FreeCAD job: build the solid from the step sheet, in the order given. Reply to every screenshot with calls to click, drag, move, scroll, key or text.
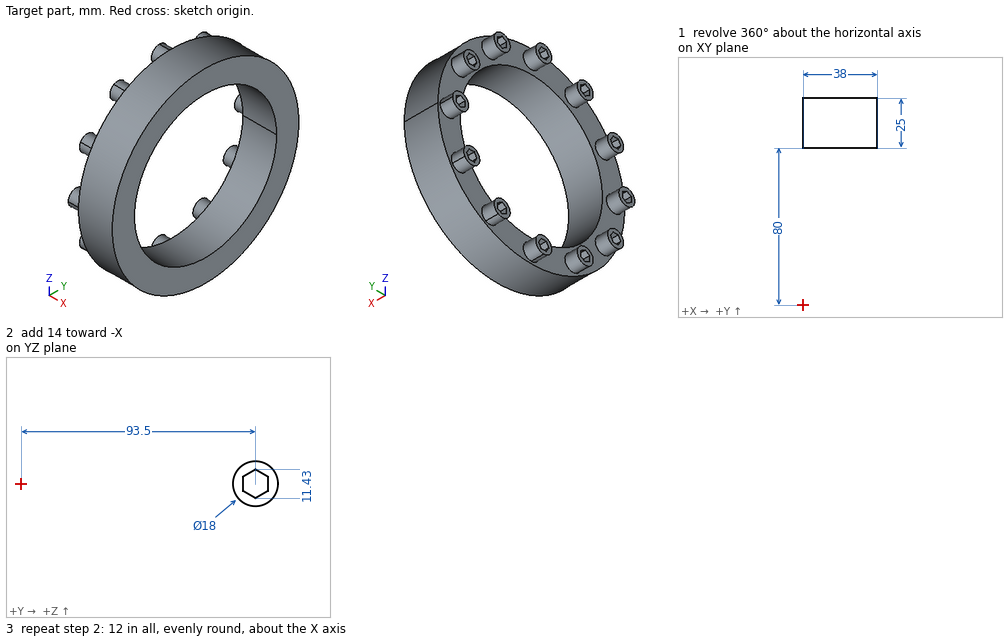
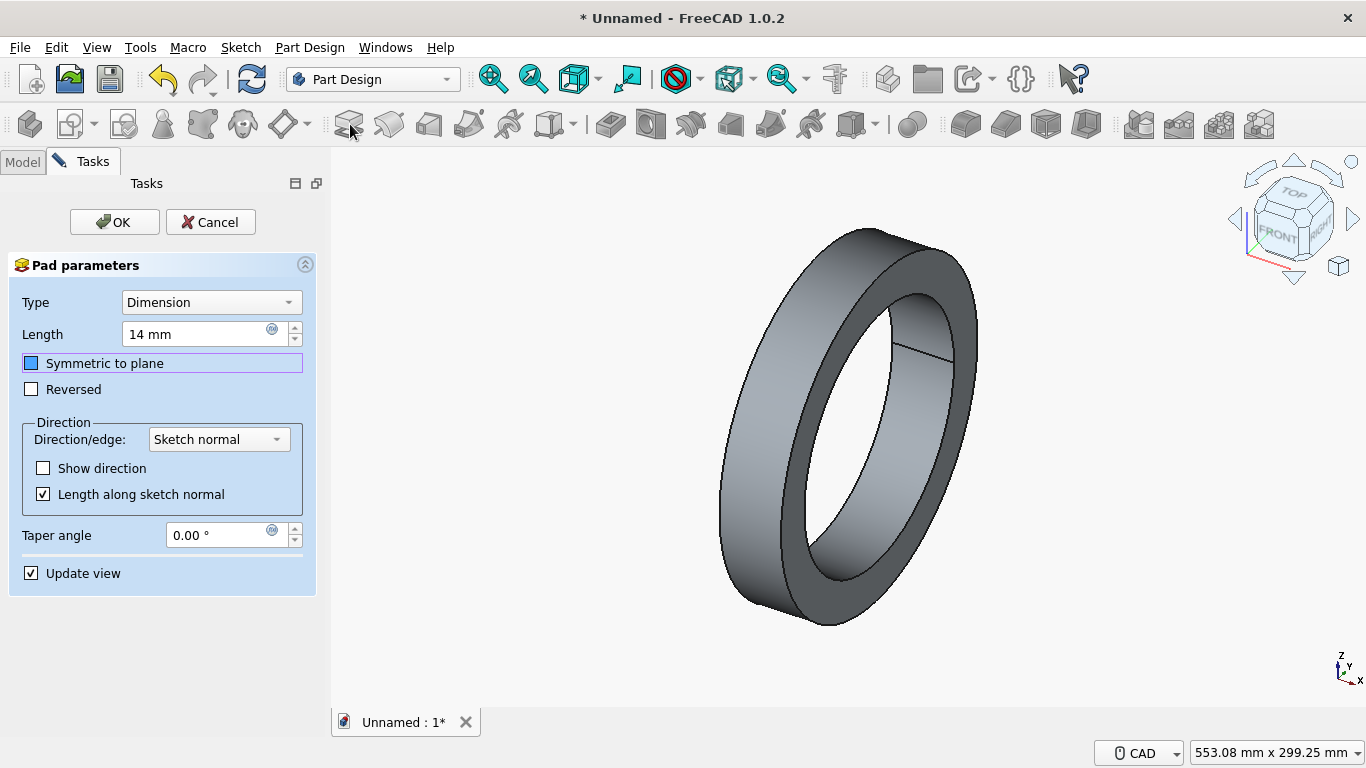
click(30, 389)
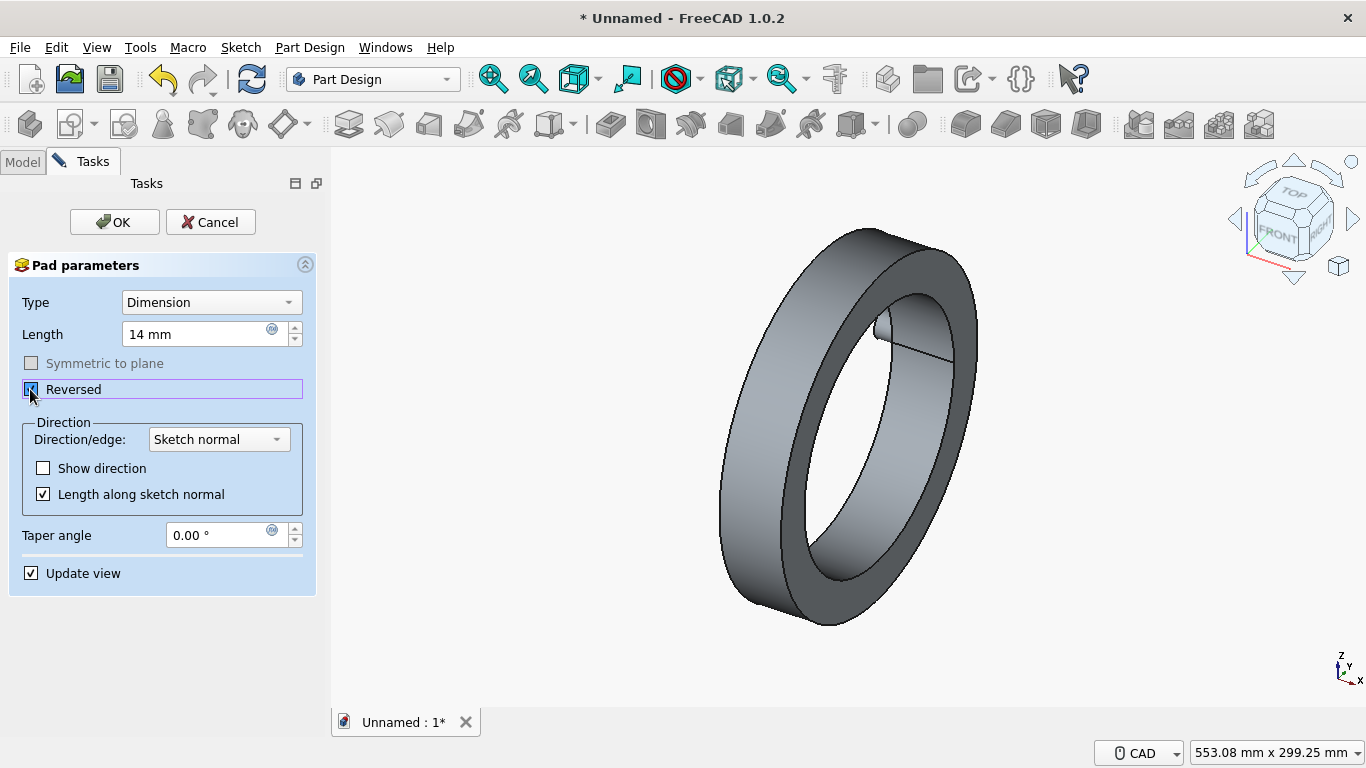
click(115, 222)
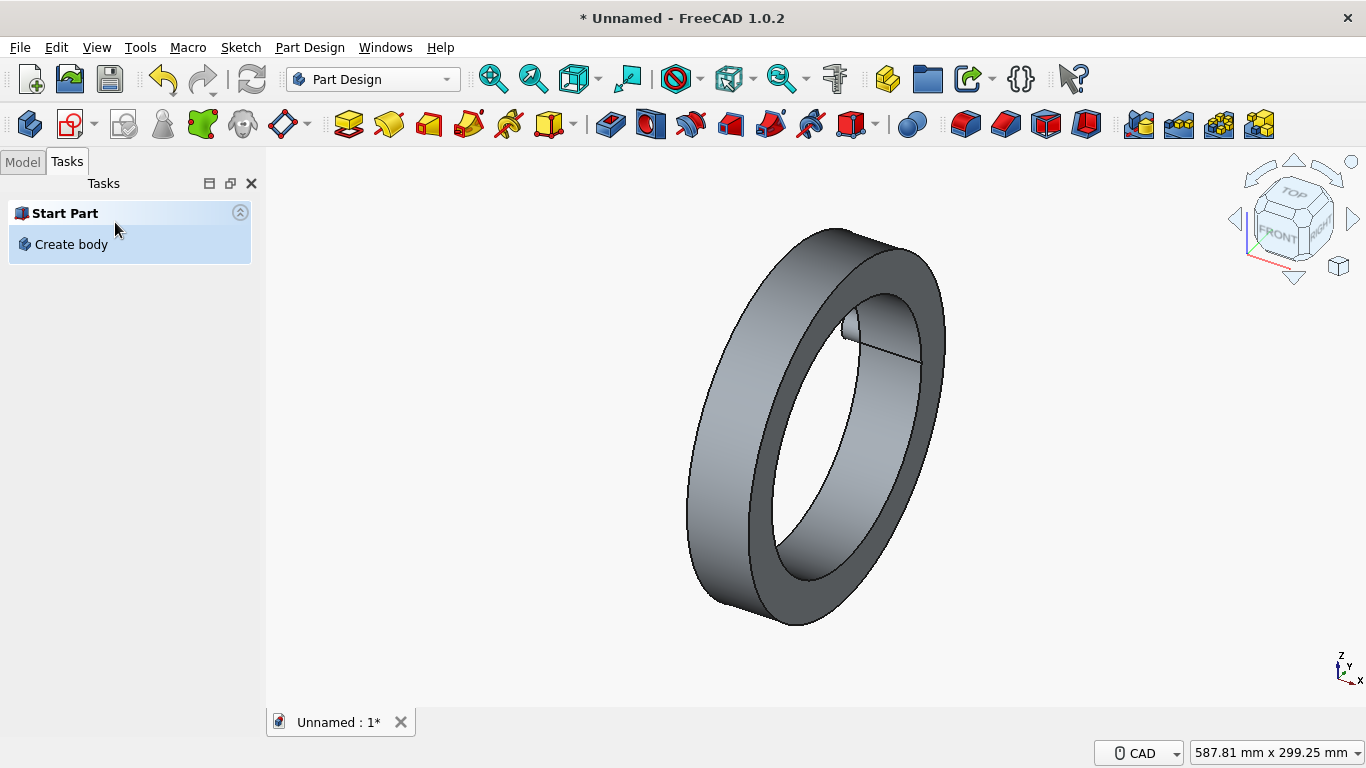
click(23, 161)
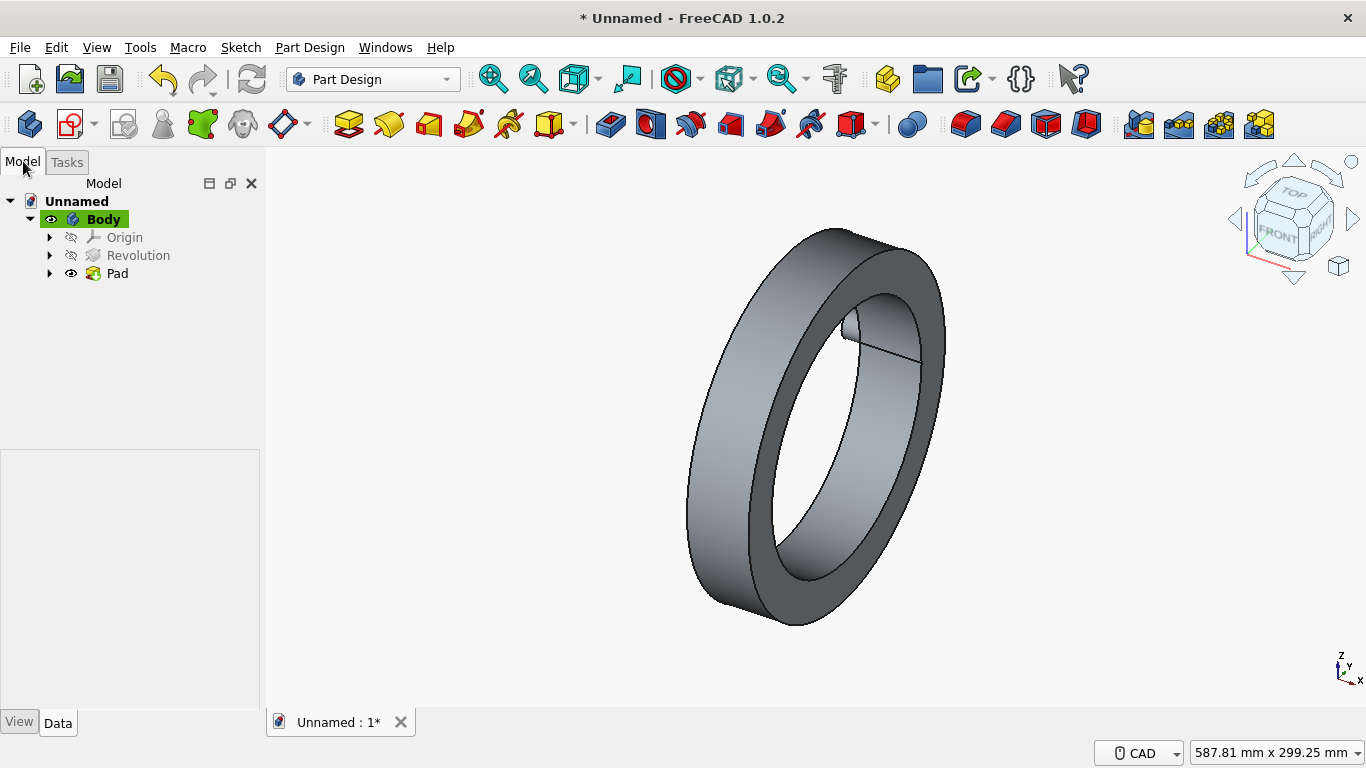
click(116, 273)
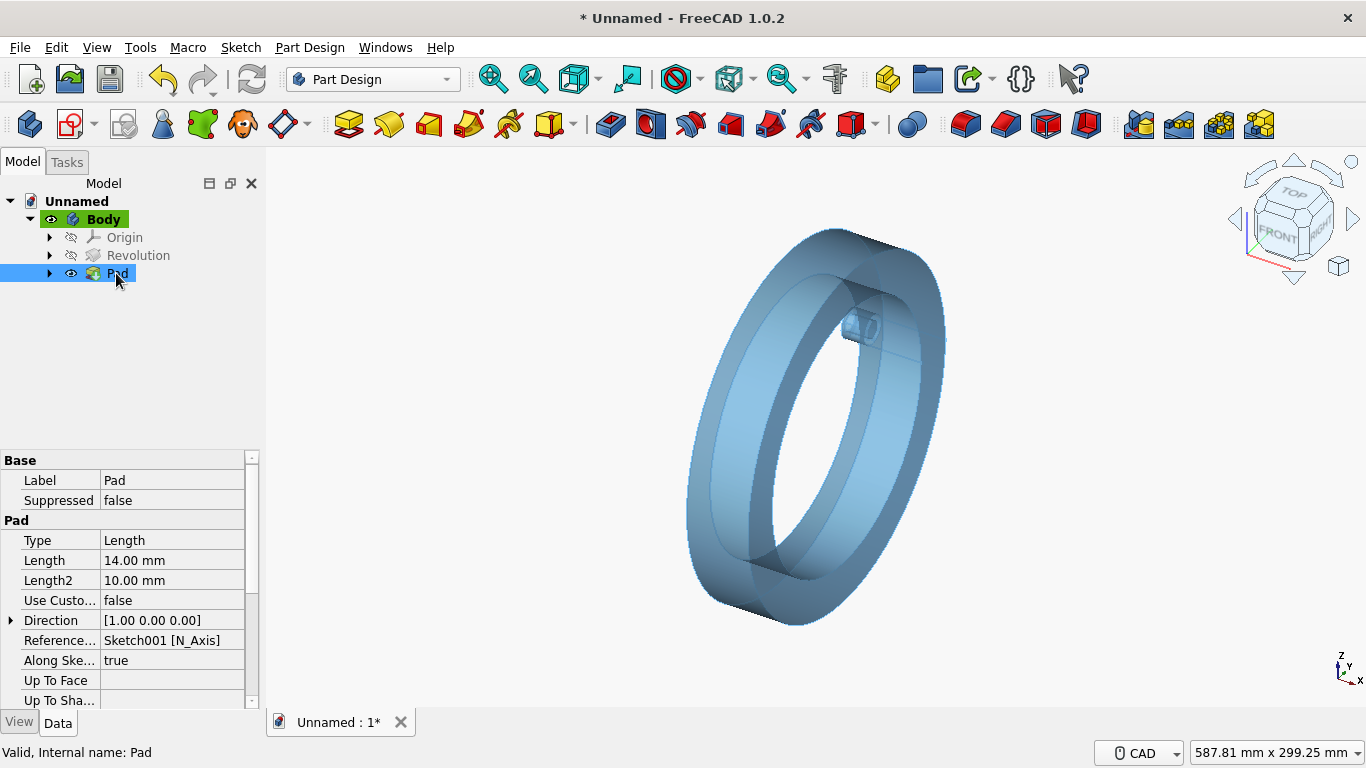
click(1220, 124)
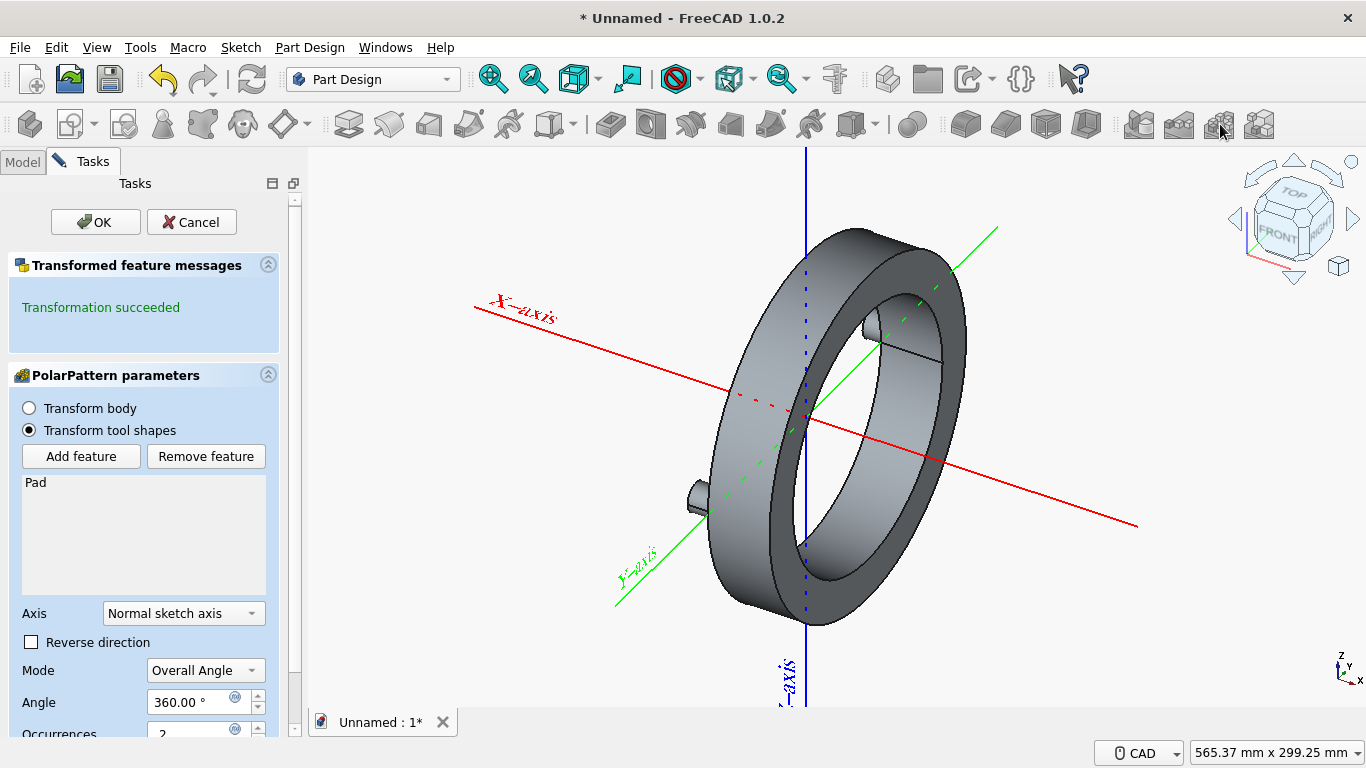
click(184, 614)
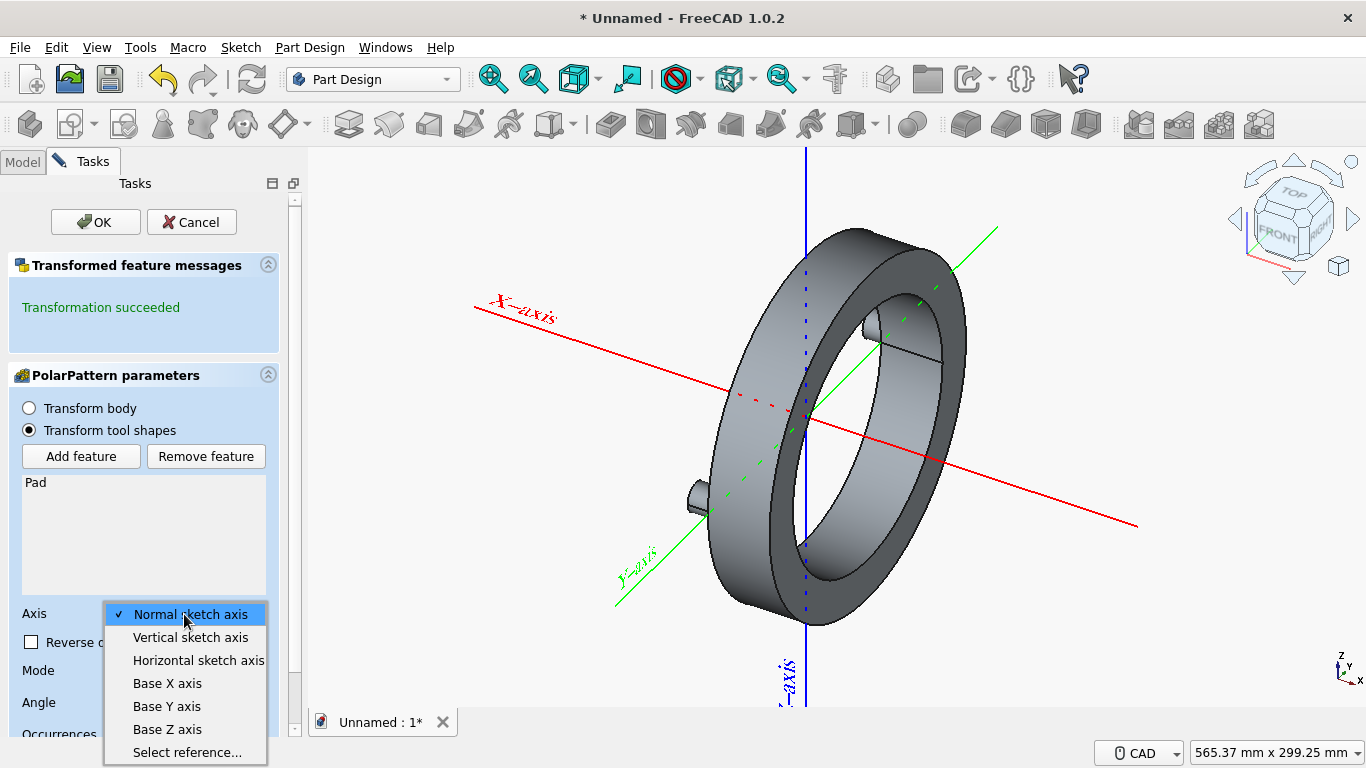
click(184, 684)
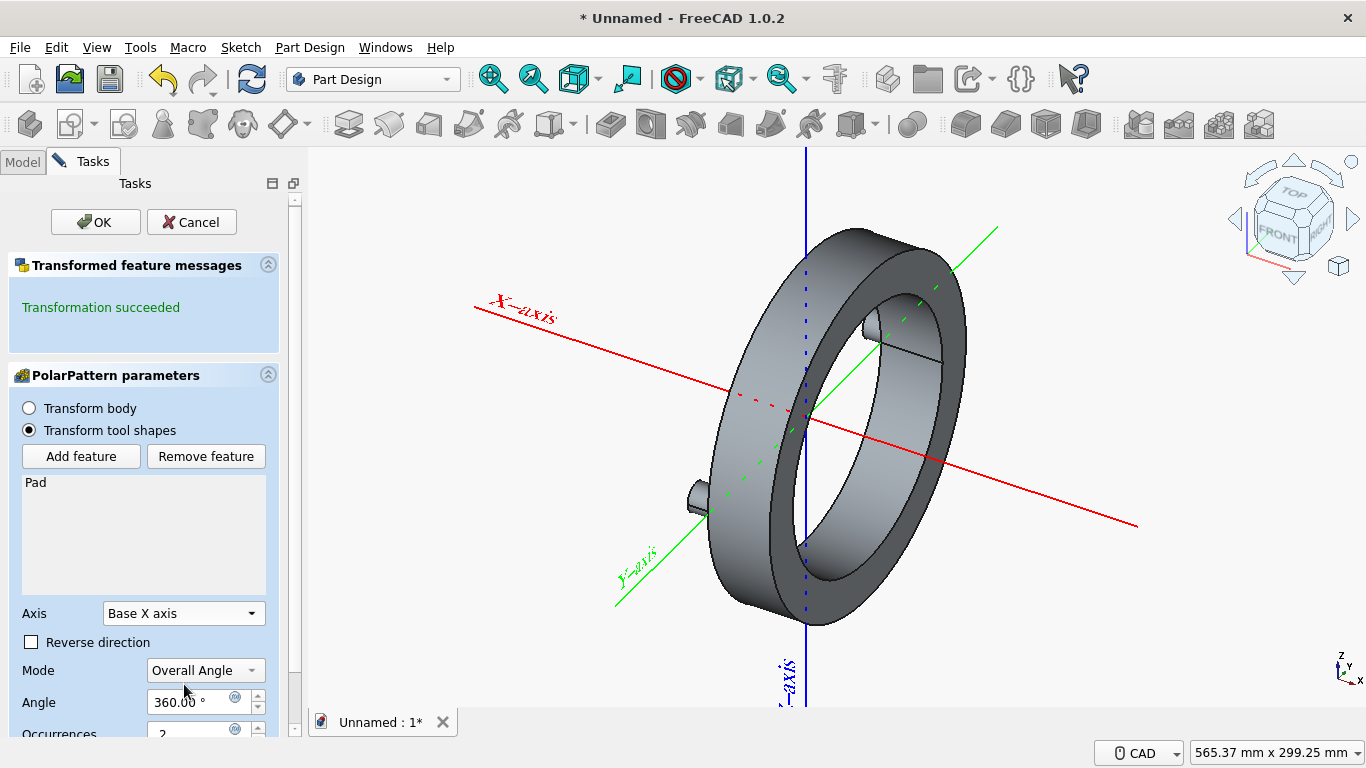
scroll(295, 464, down, 2)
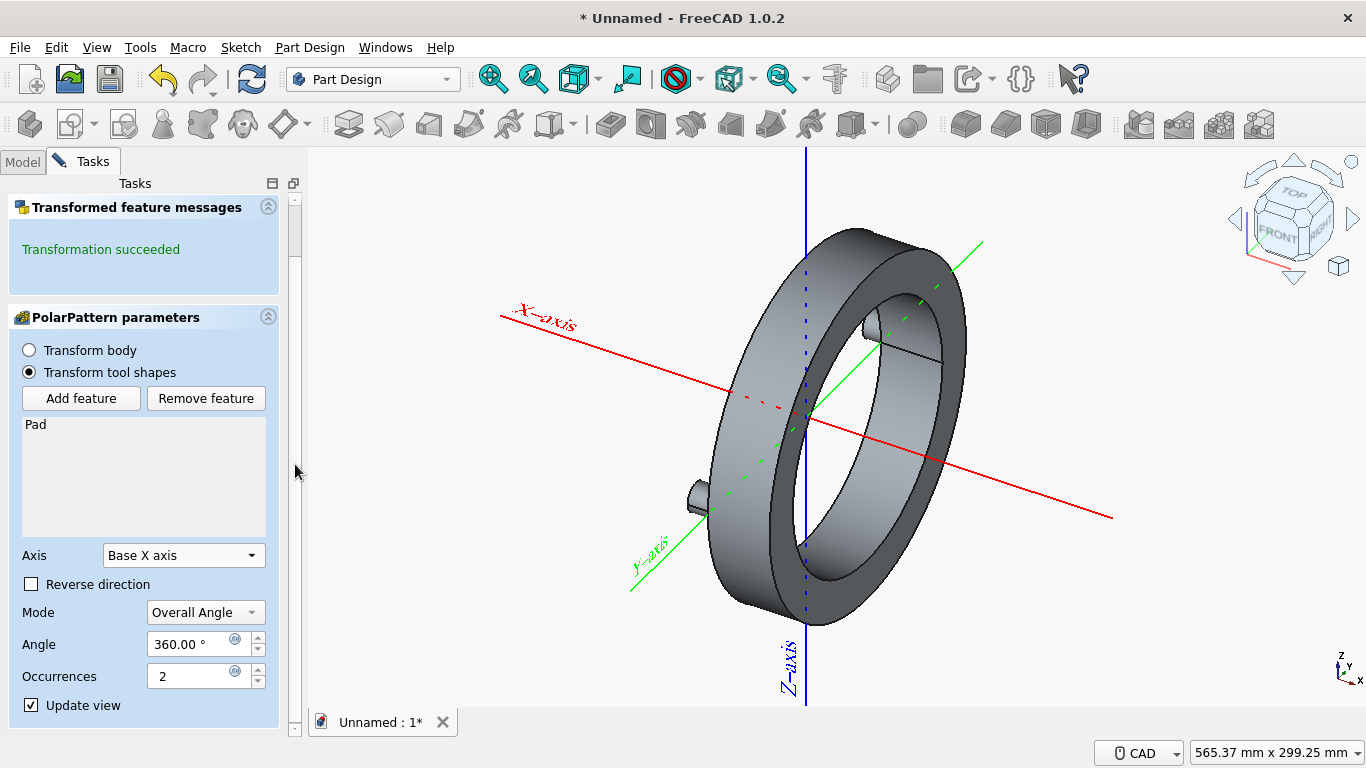
triple_click(198, 676)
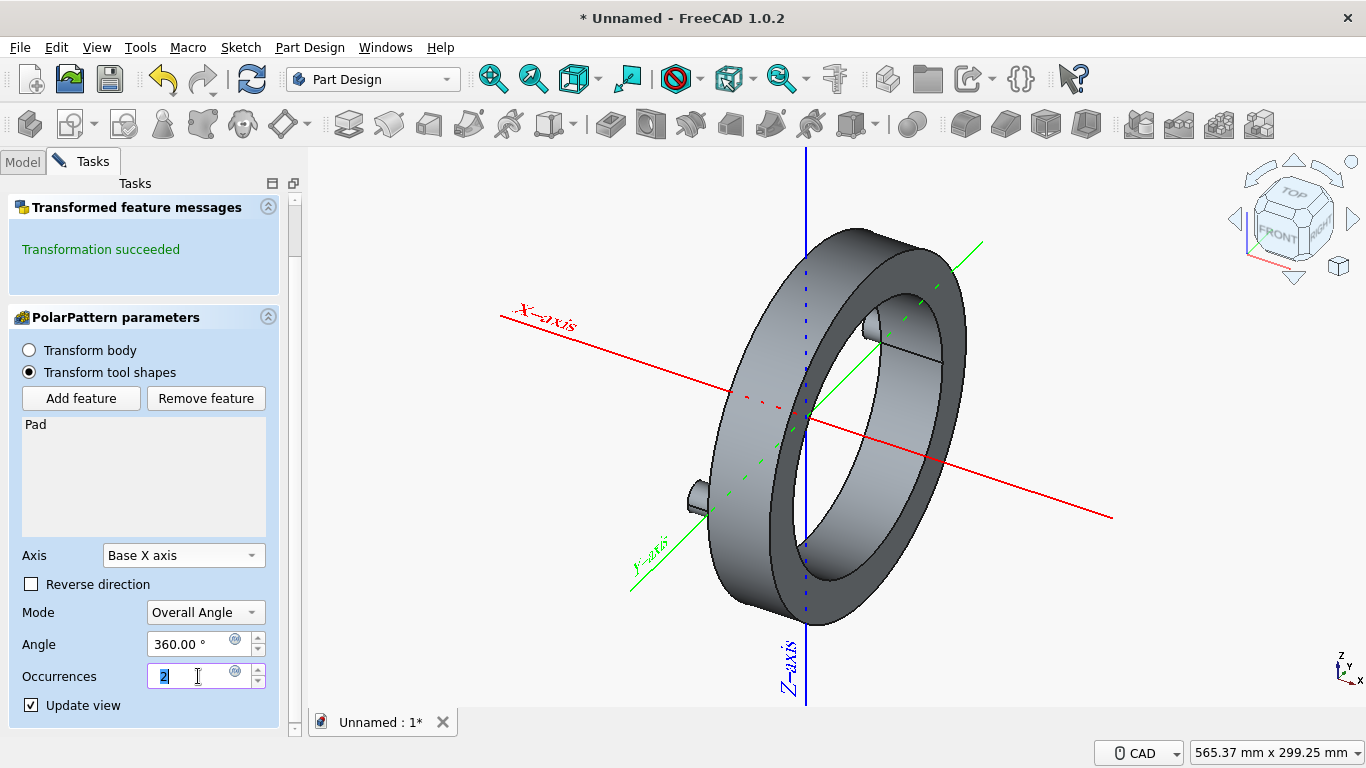
text(12)
key(Tab)